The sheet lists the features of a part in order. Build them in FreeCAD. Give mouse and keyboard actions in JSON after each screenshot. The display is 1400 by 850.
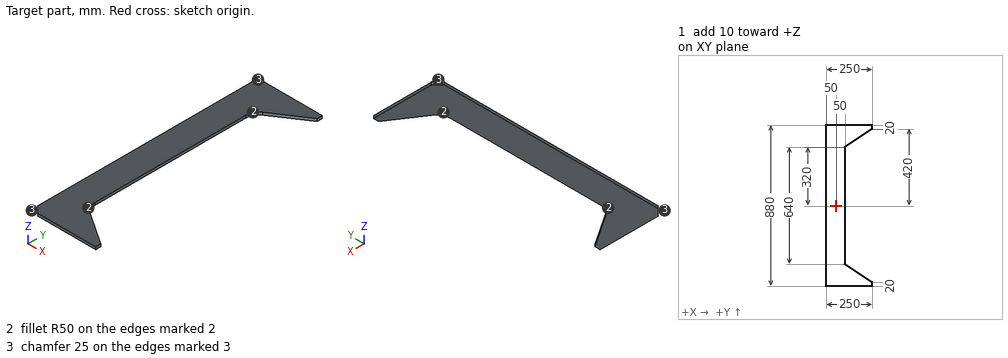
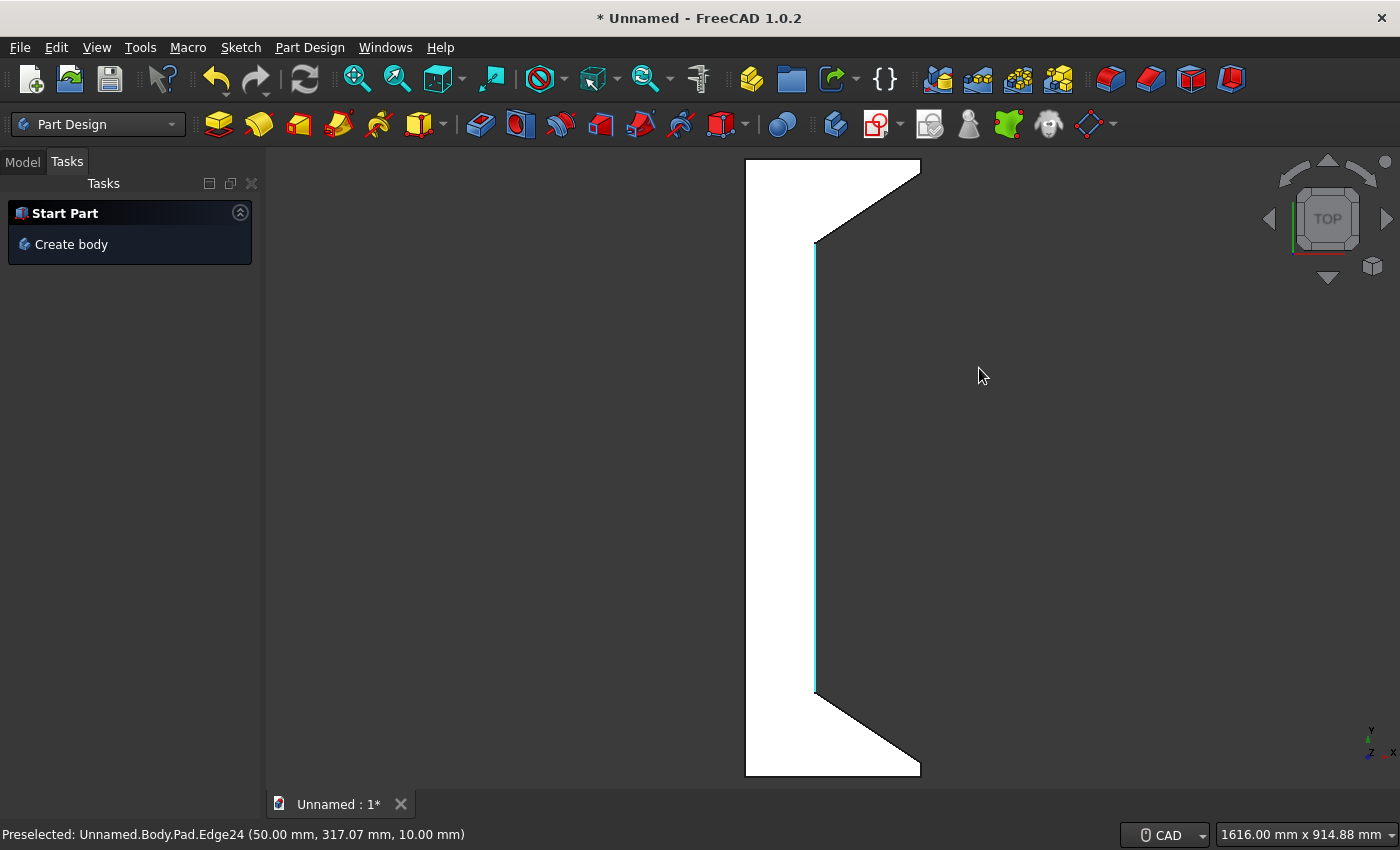
{"action": "scroll", "coordinate": [815, 242], "scroll_direction": "up", "scroll_amount": 9}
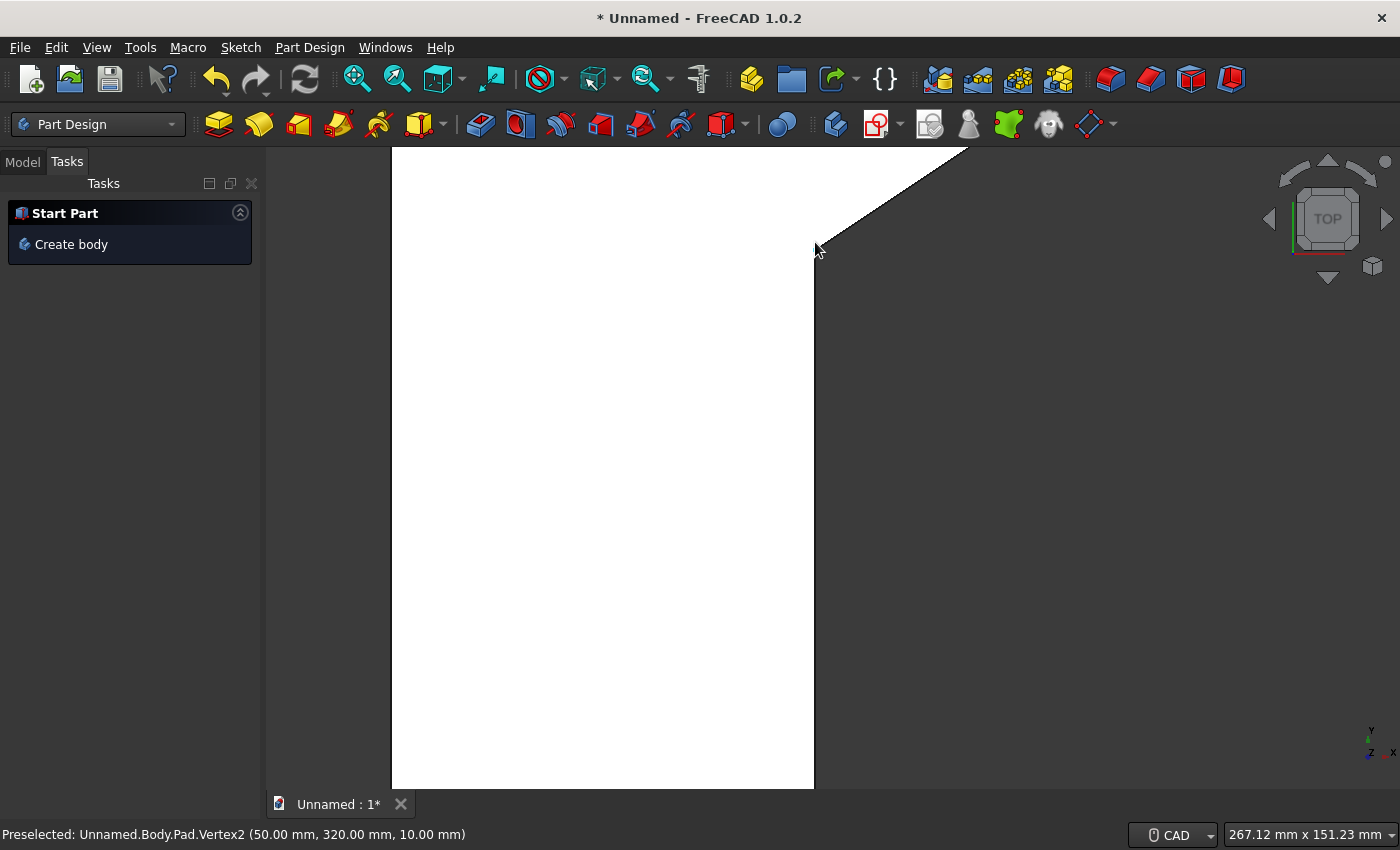
{"action": "left_click", "coordinate": [358, 80]}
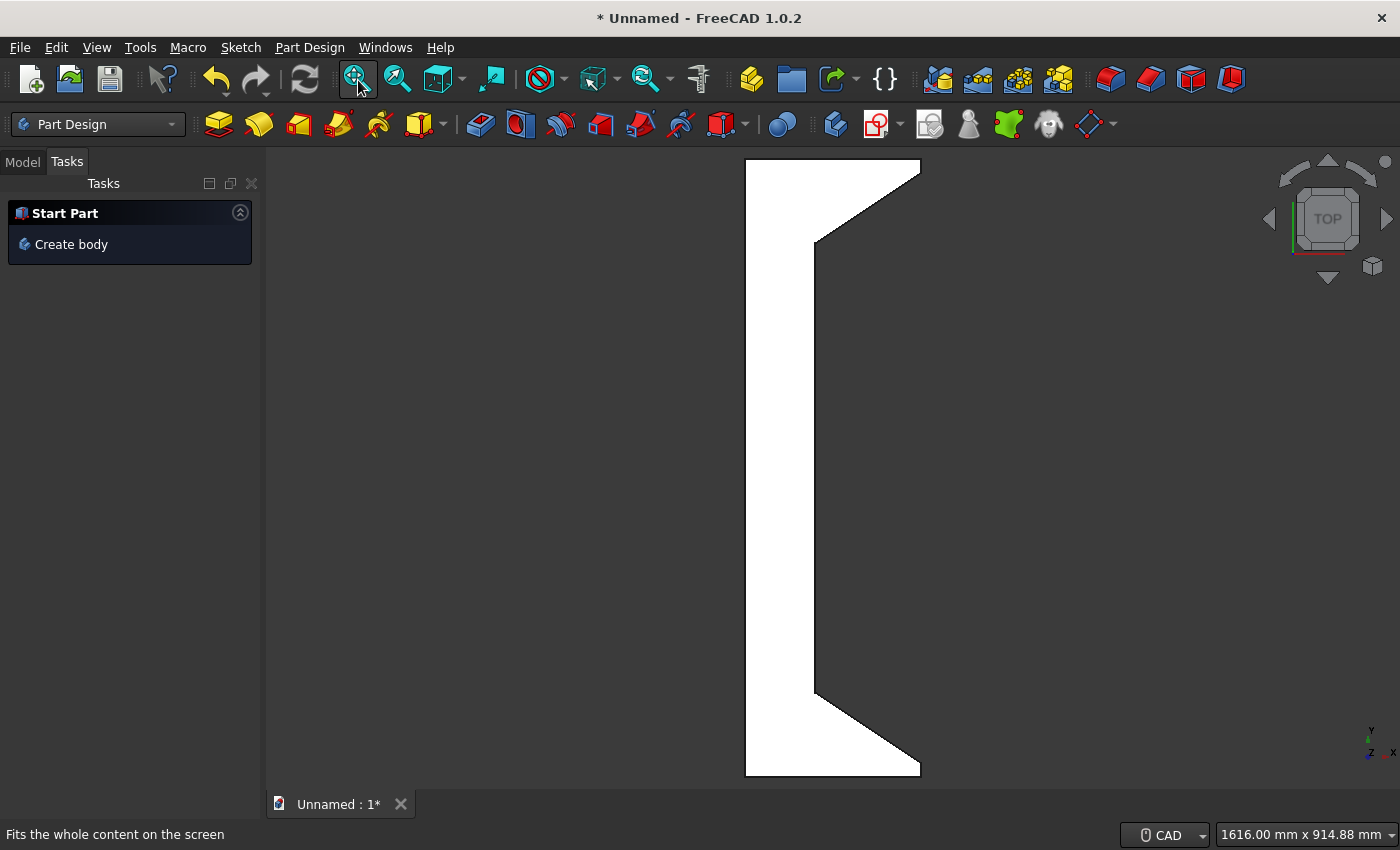
{"action": "key", "text": "1"}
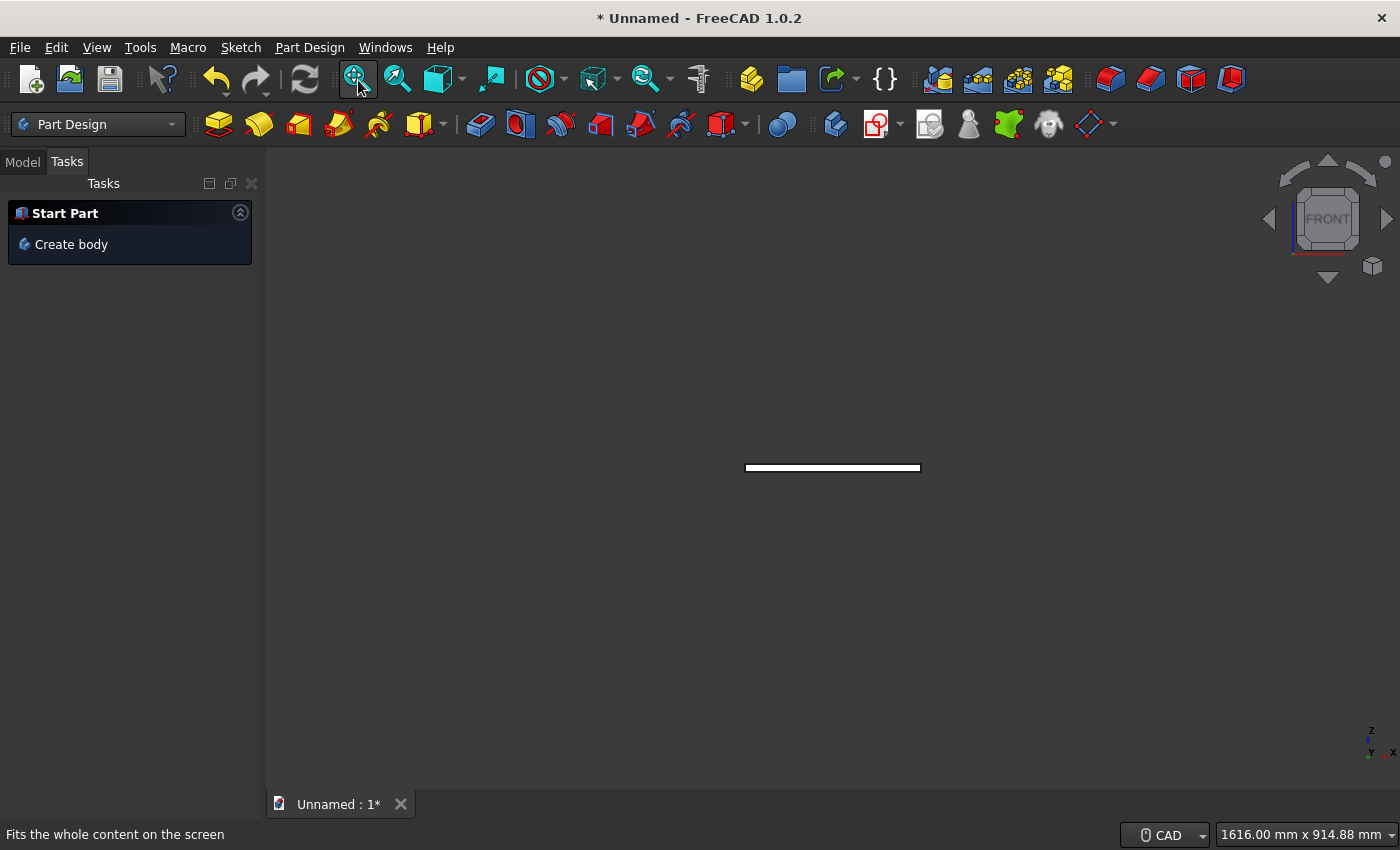
{"action": "key", "text": "v f"}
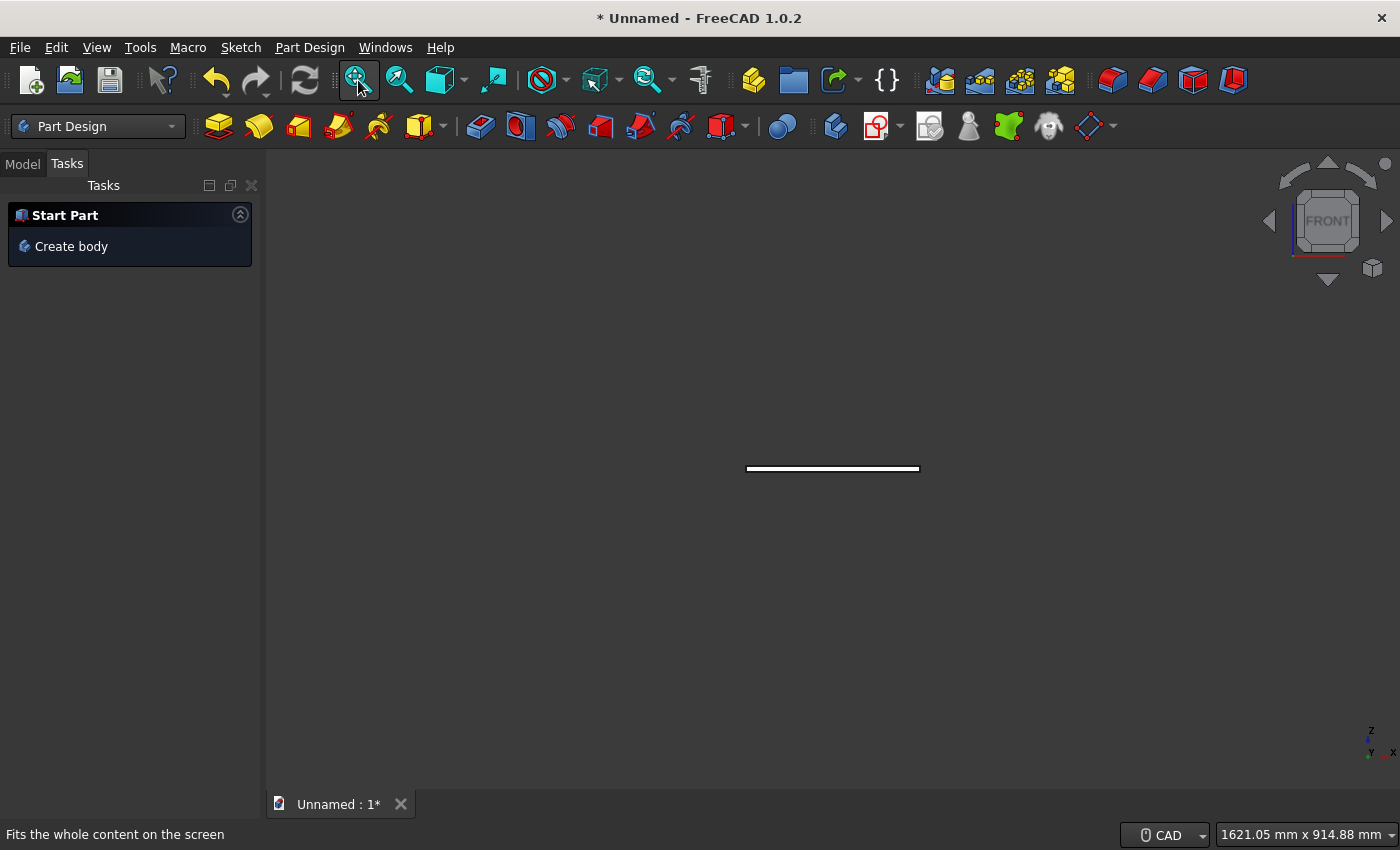
{"action": "scroll", "coordinate": [816, 468], "scroll_direction": "up", "scroll_amount": 9}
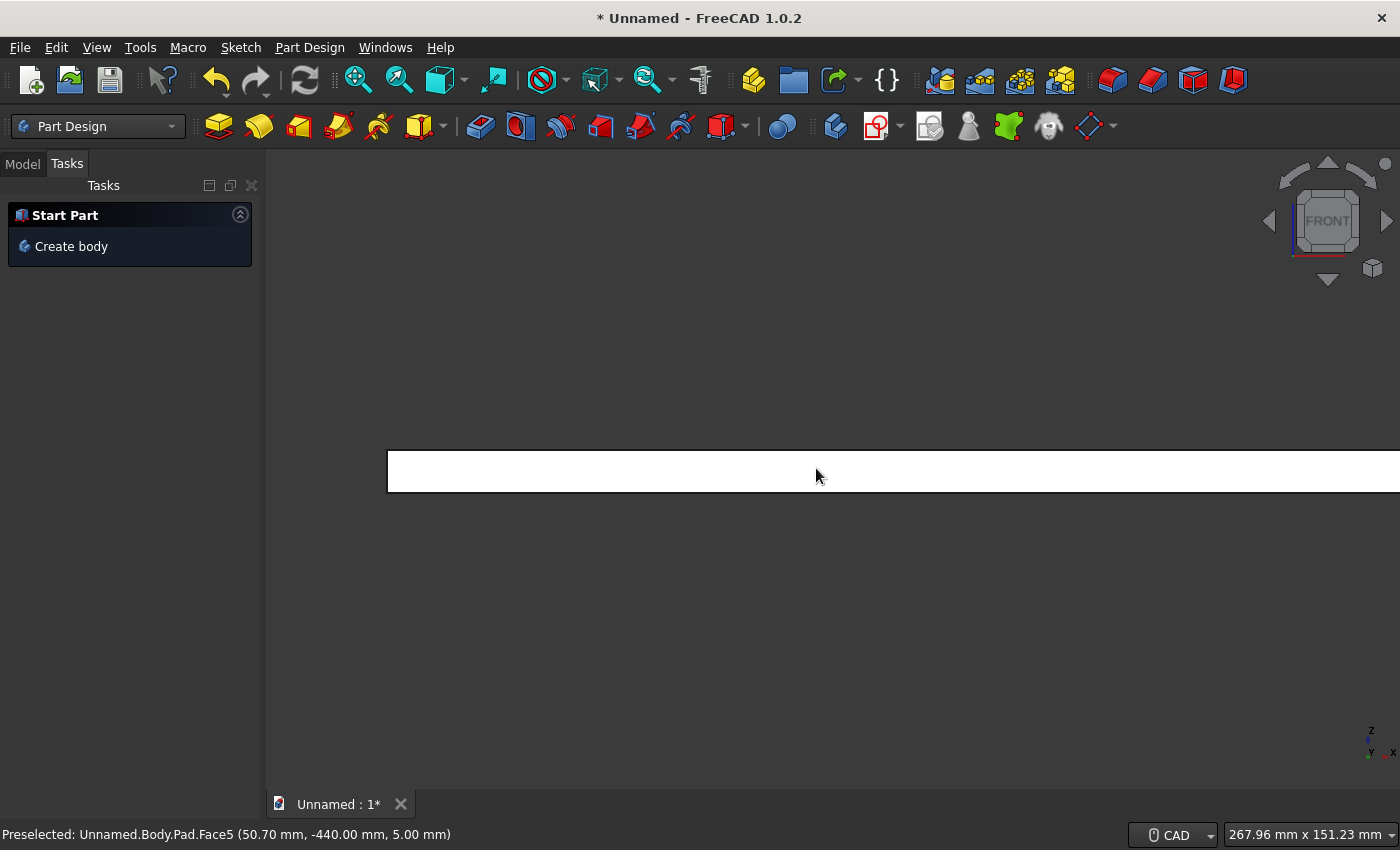
{"action": "key", "text": "v f"}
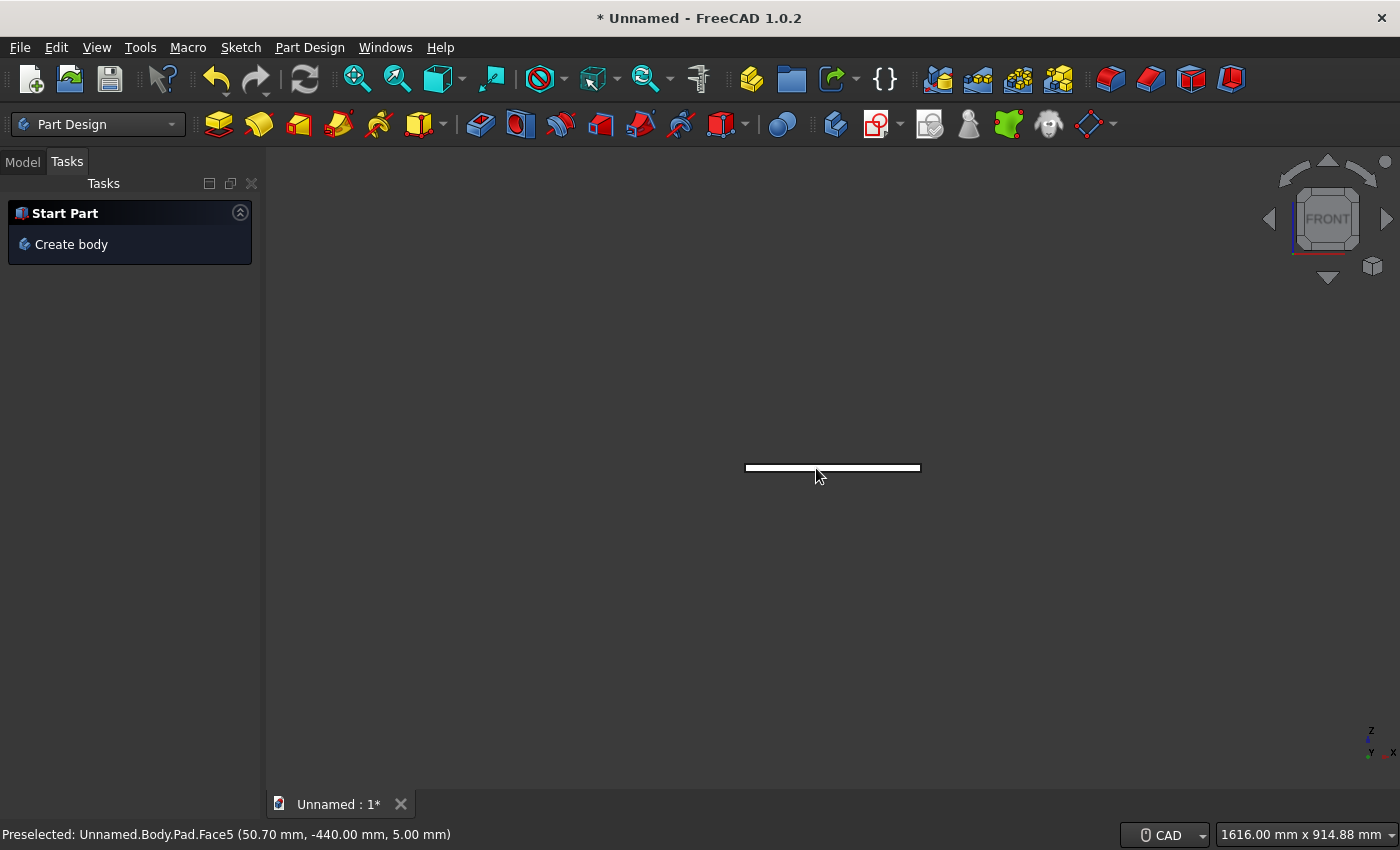
{"action": "key", "text": "3"}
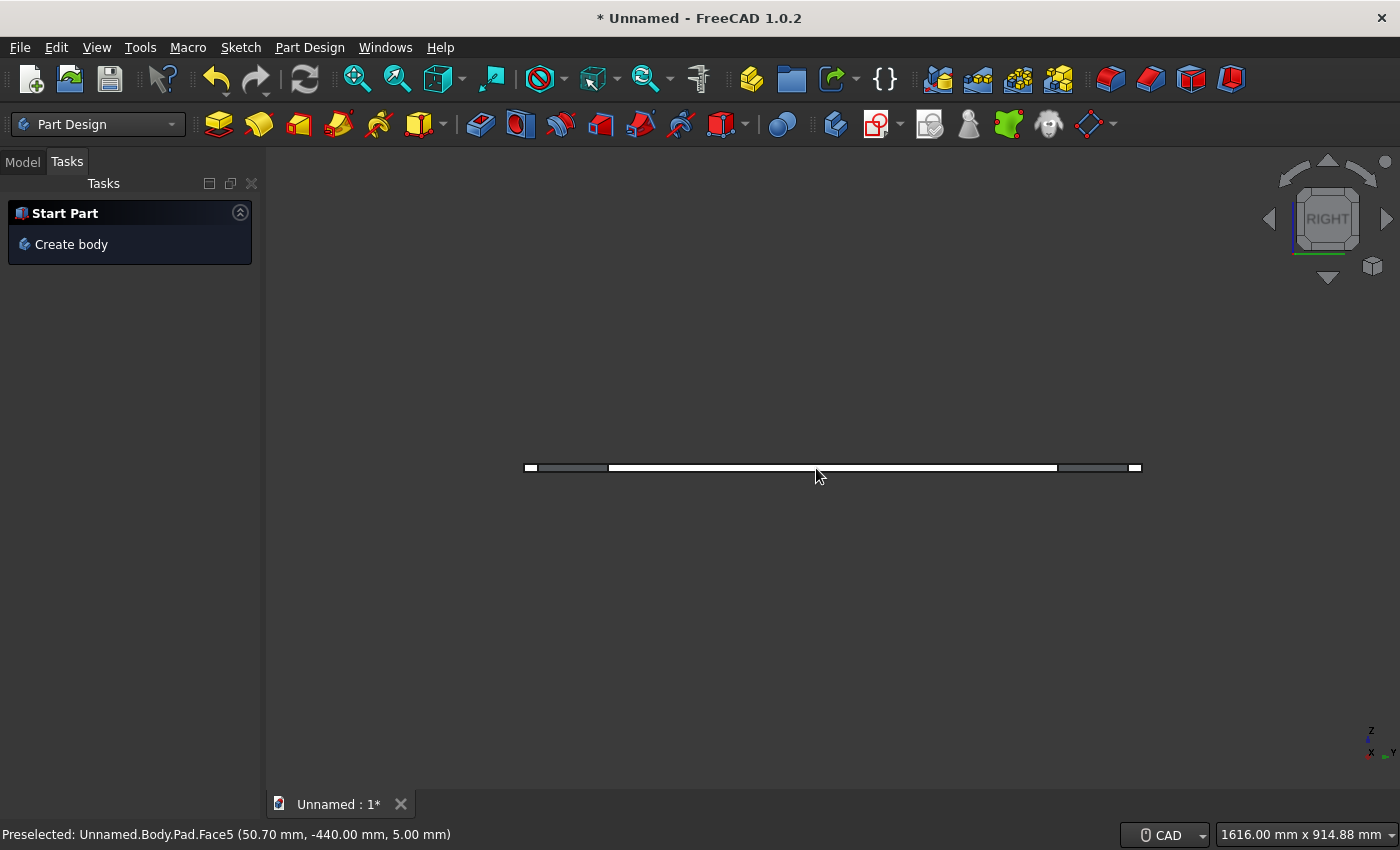
{"action": "scroll", "coordinate": [1058, 467], "scroll_direction": "up", "scroll_amount": 9}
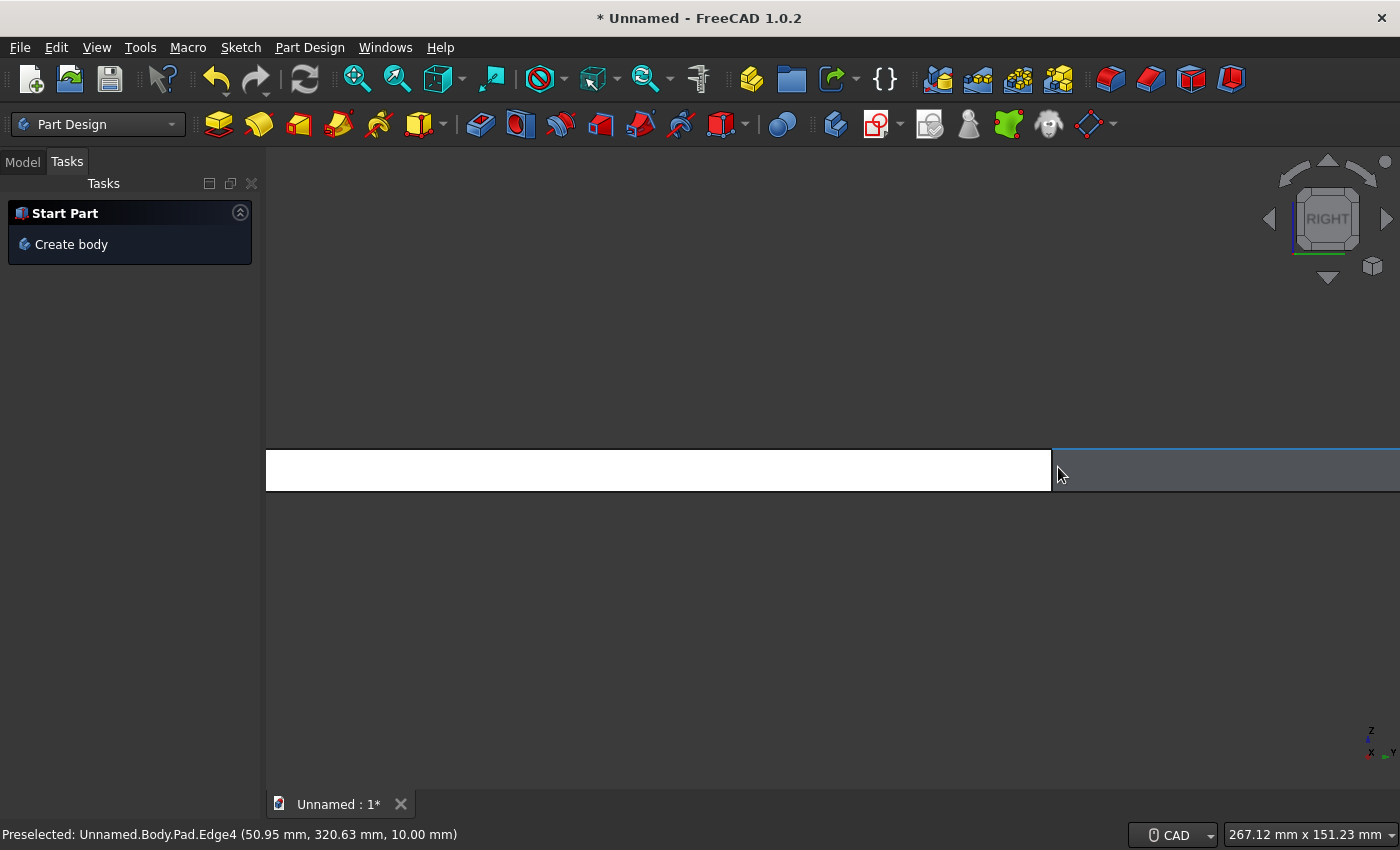
{"action": "left_click", "coordinate": [358, 80]}